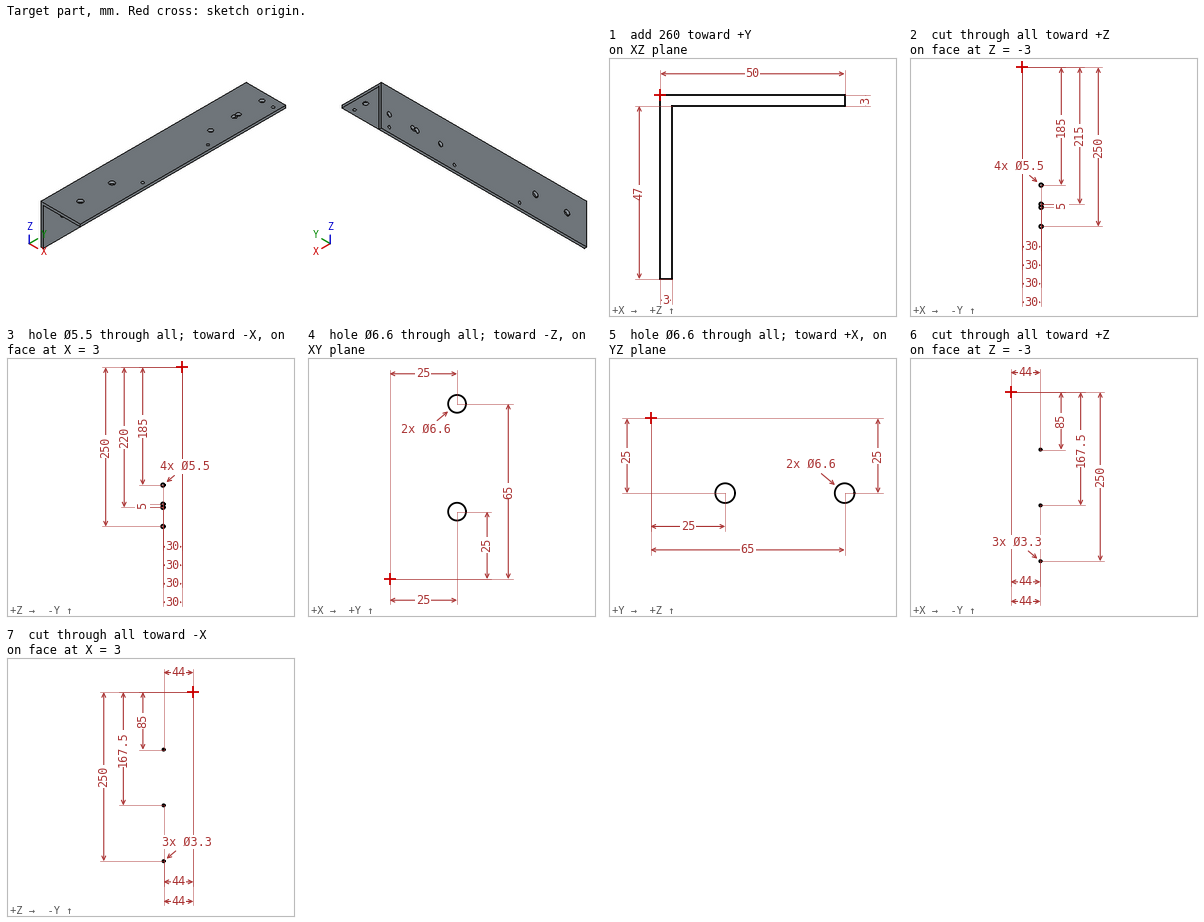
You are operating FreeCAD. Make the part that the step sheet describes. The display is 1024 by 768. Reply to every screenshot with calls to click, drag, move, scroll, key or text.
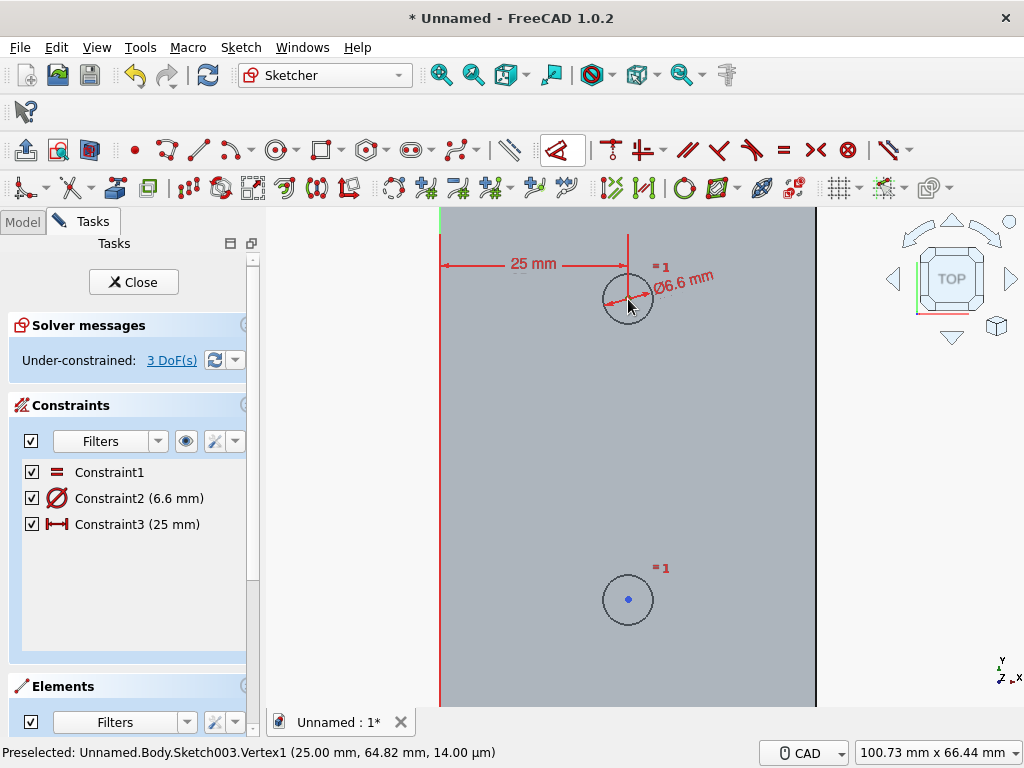
key(i)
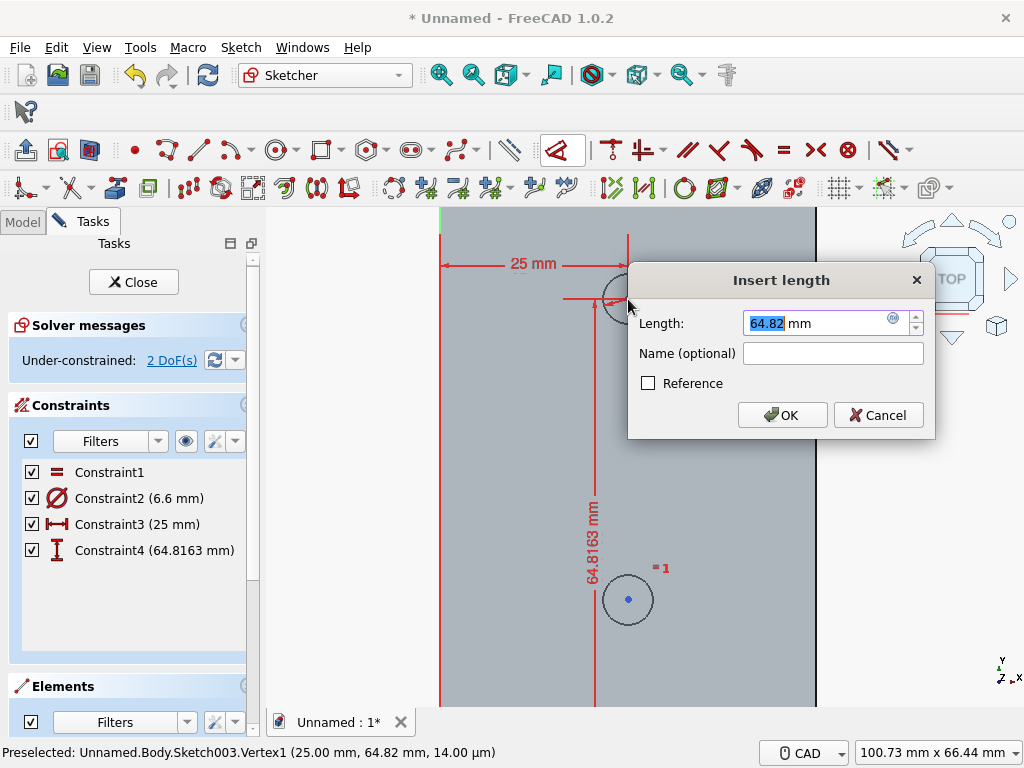
text(65)
key(Return)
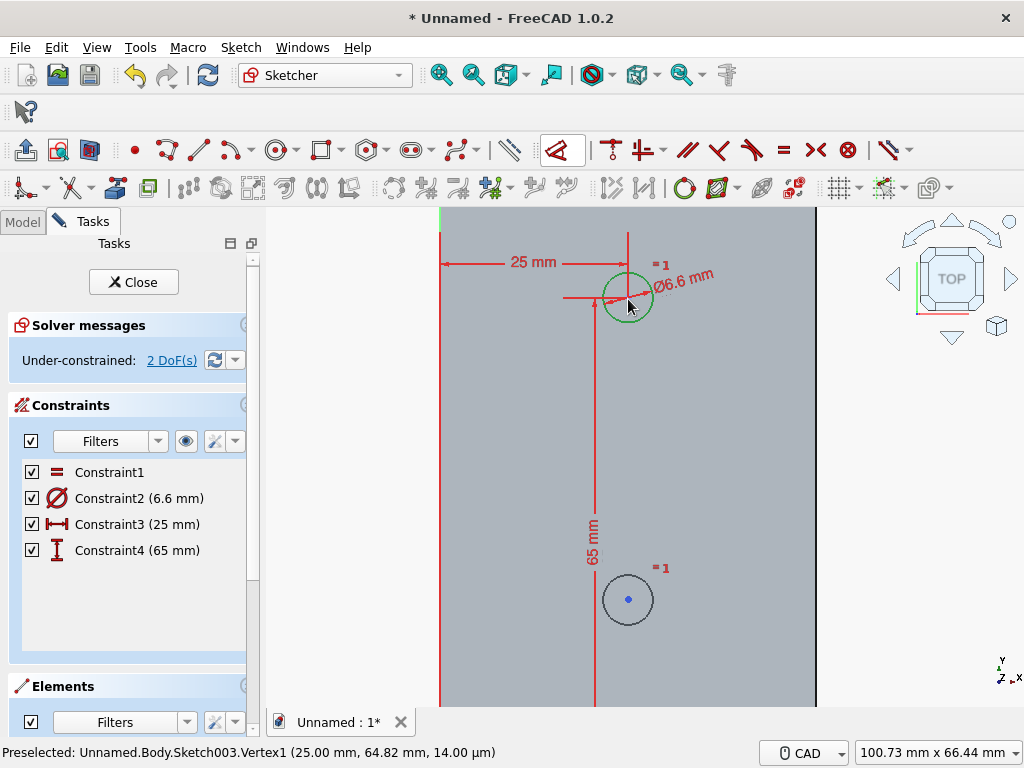
click(628, 600)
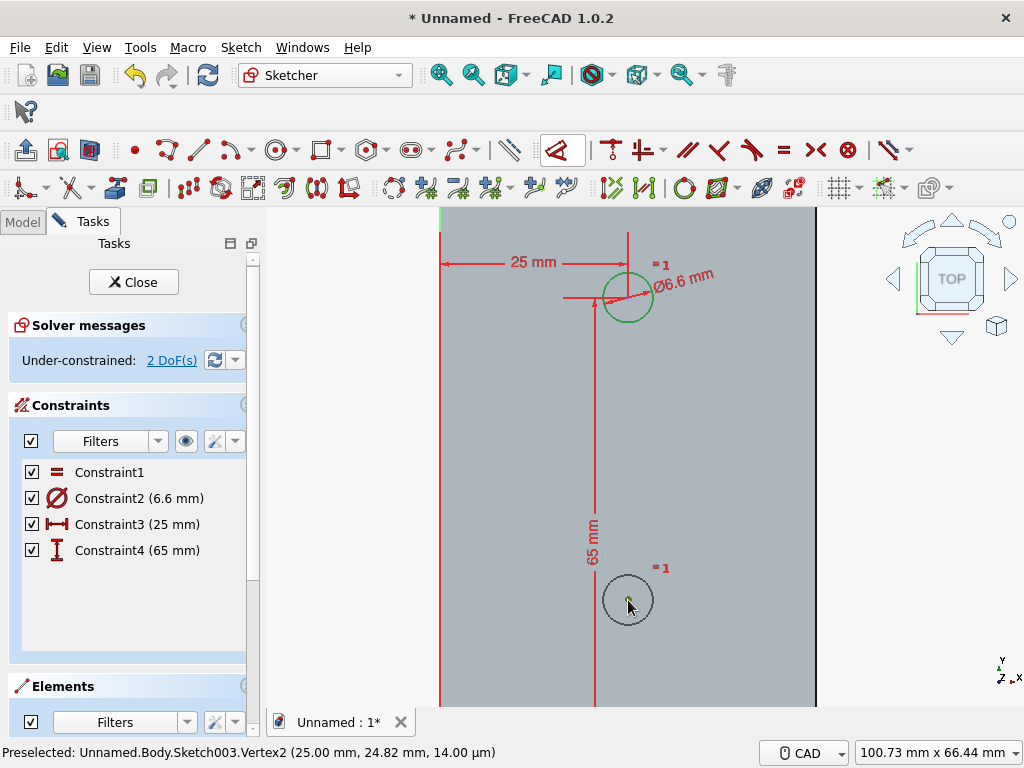
key(l)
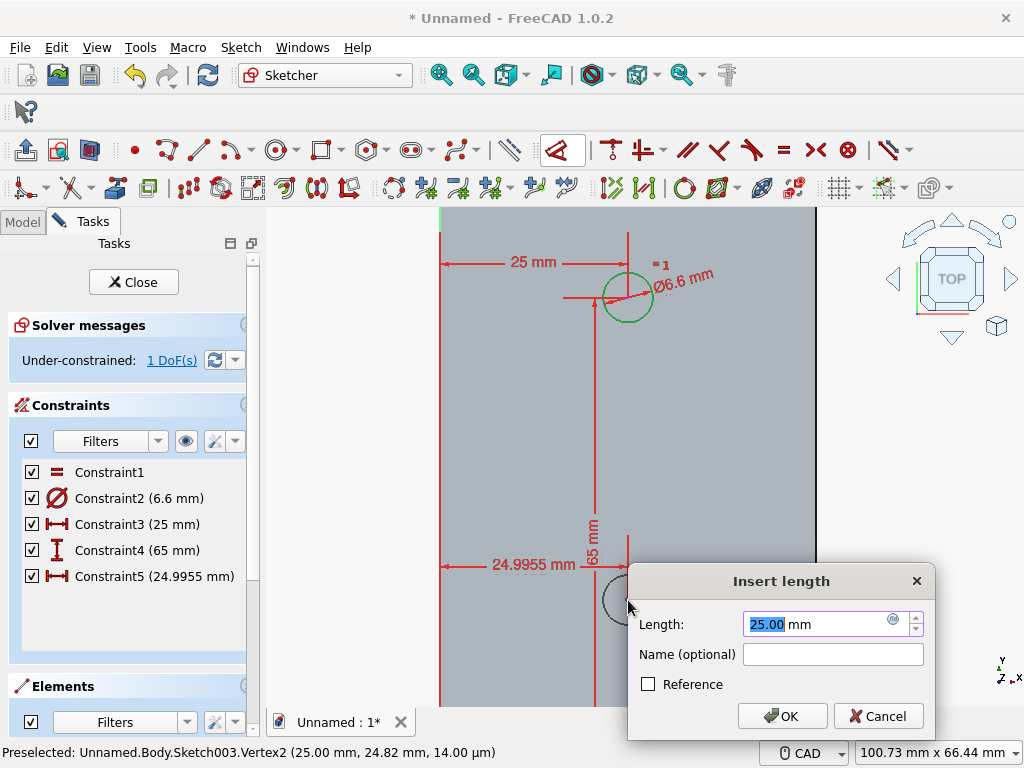
text(25)
key(Return)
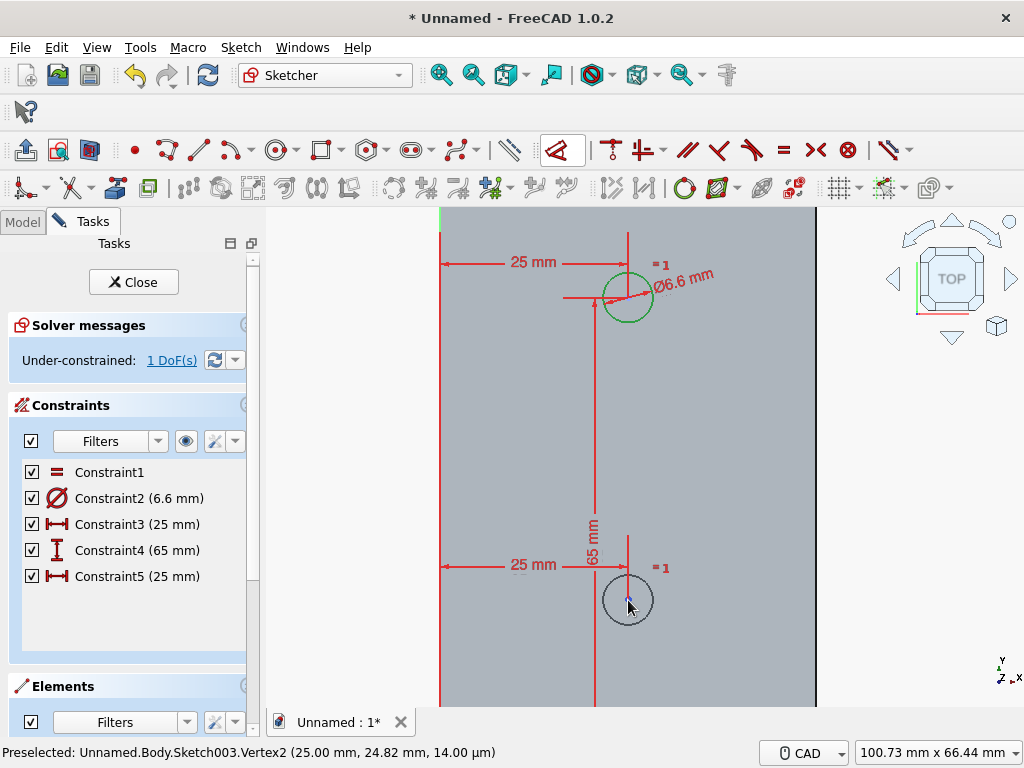
click(628, 600)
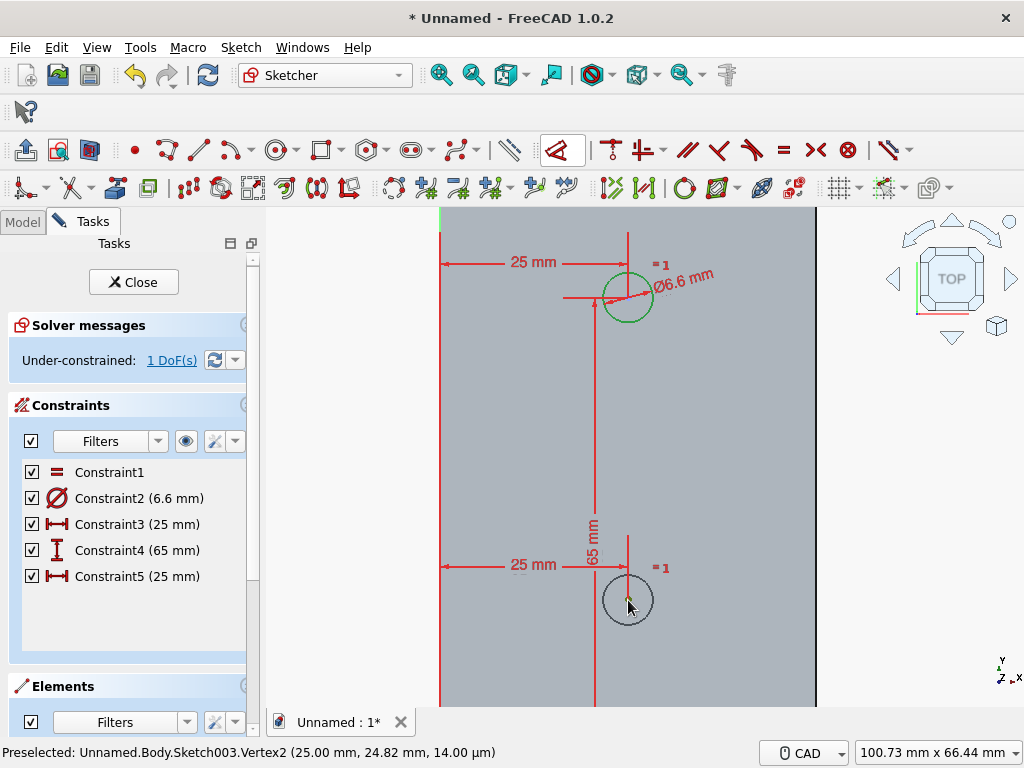
key(i)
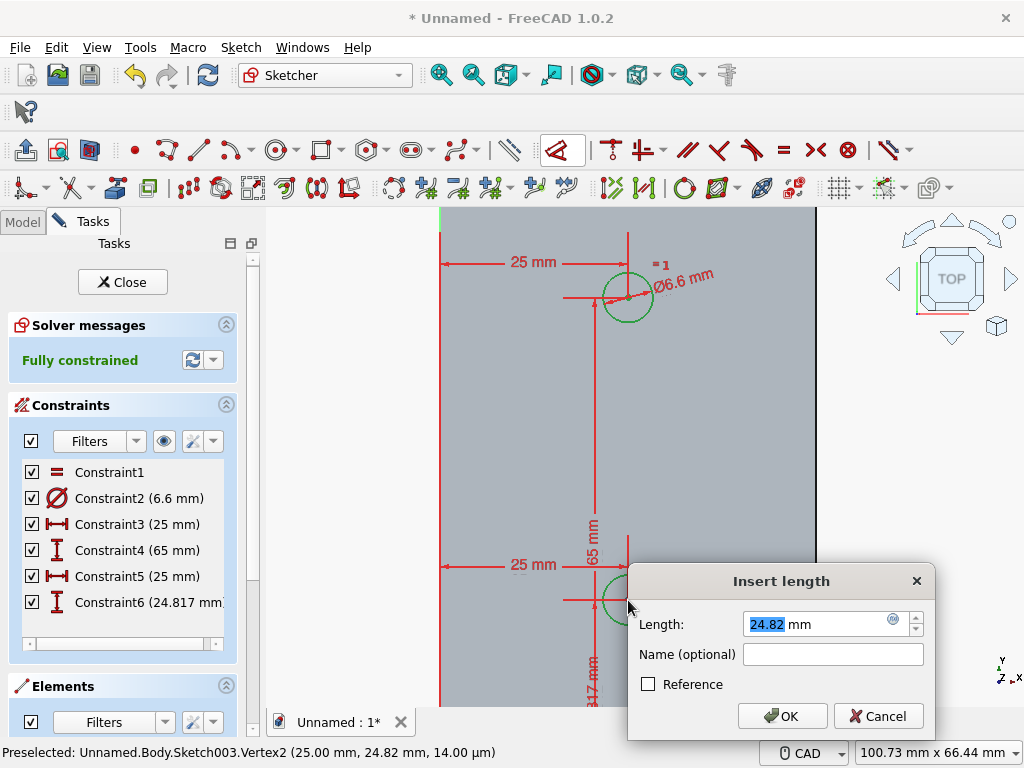
text(25)
key(Return)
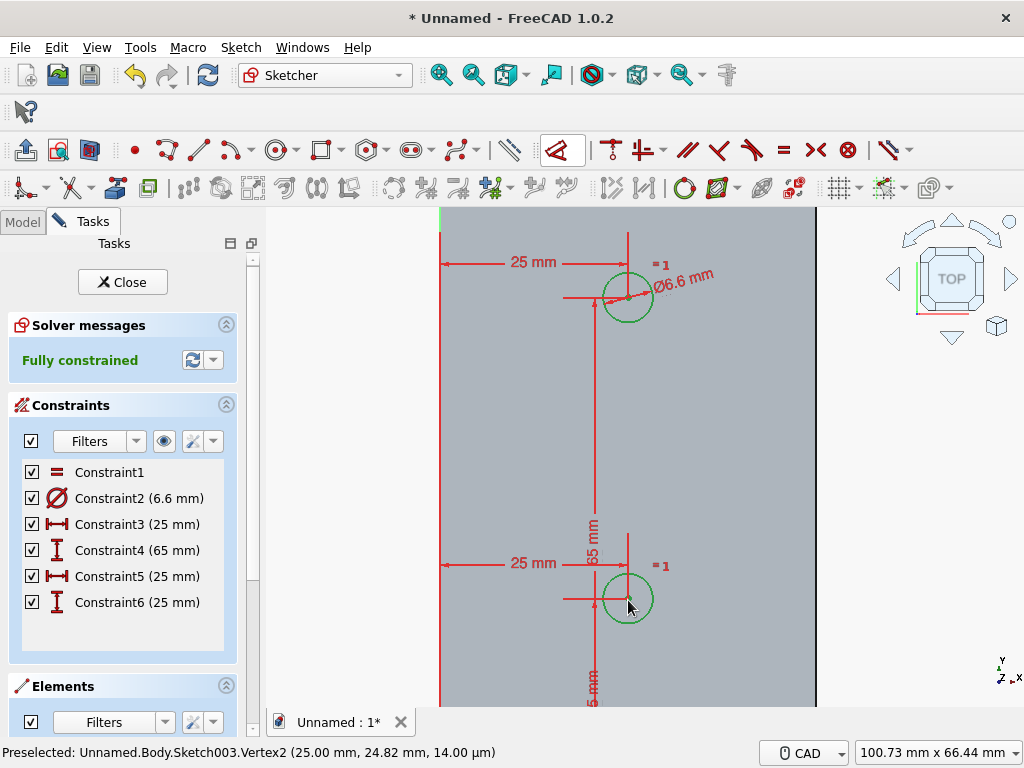
click(123, 282)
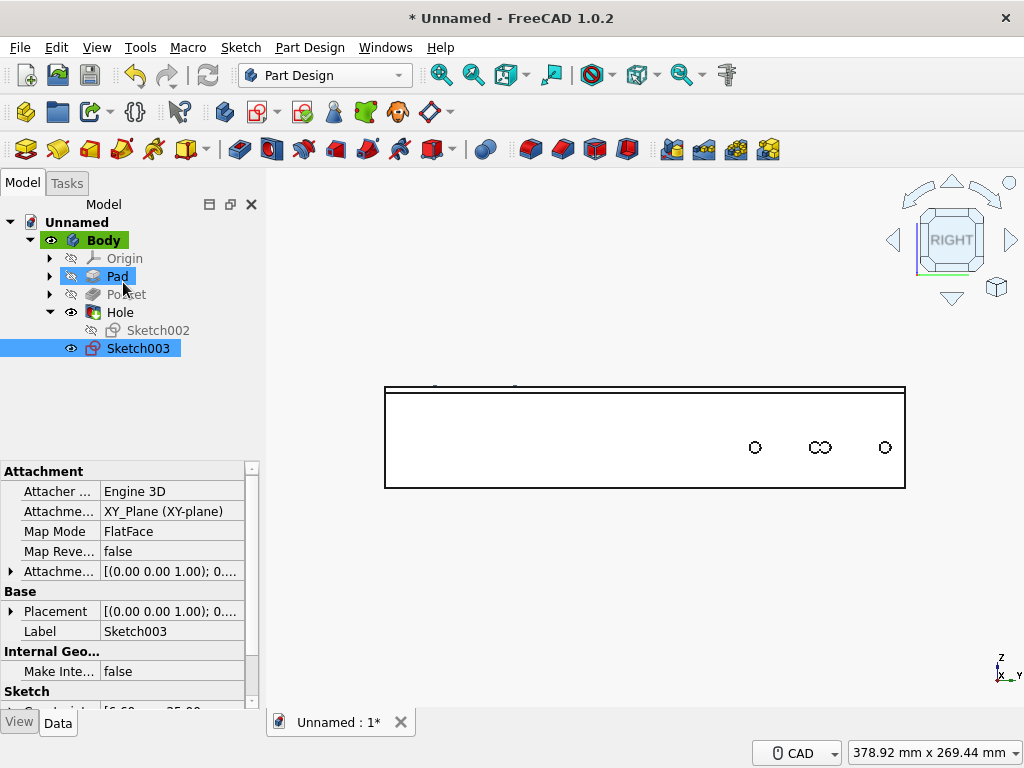
click(272, 150)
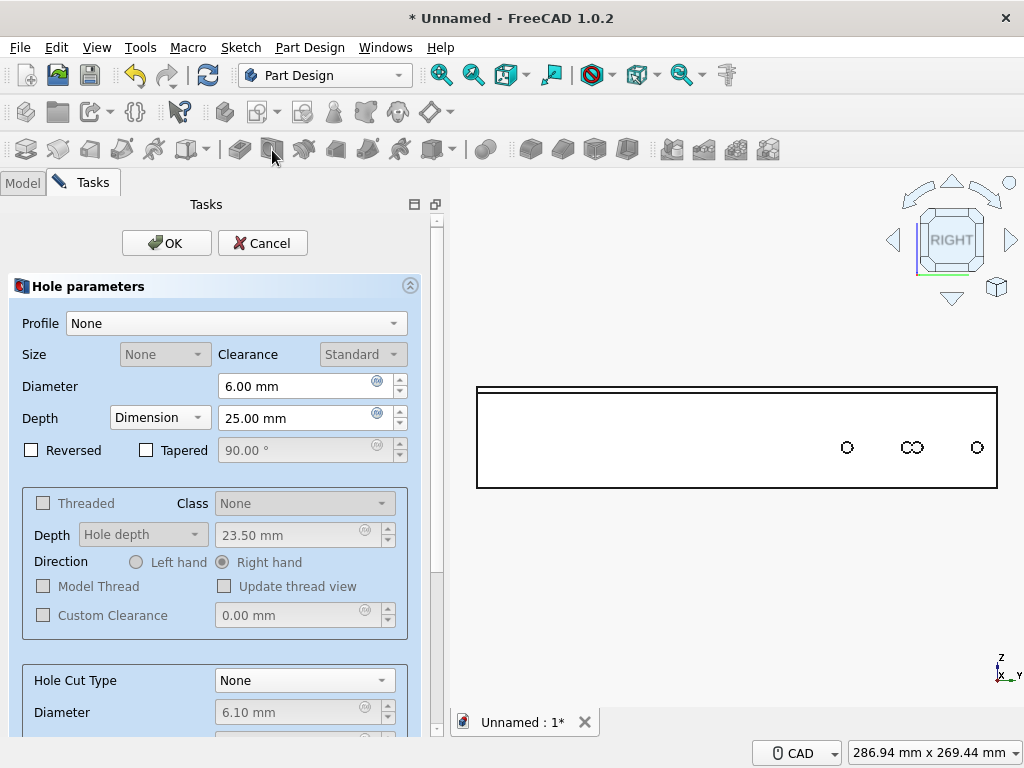
triple_click(305, 386)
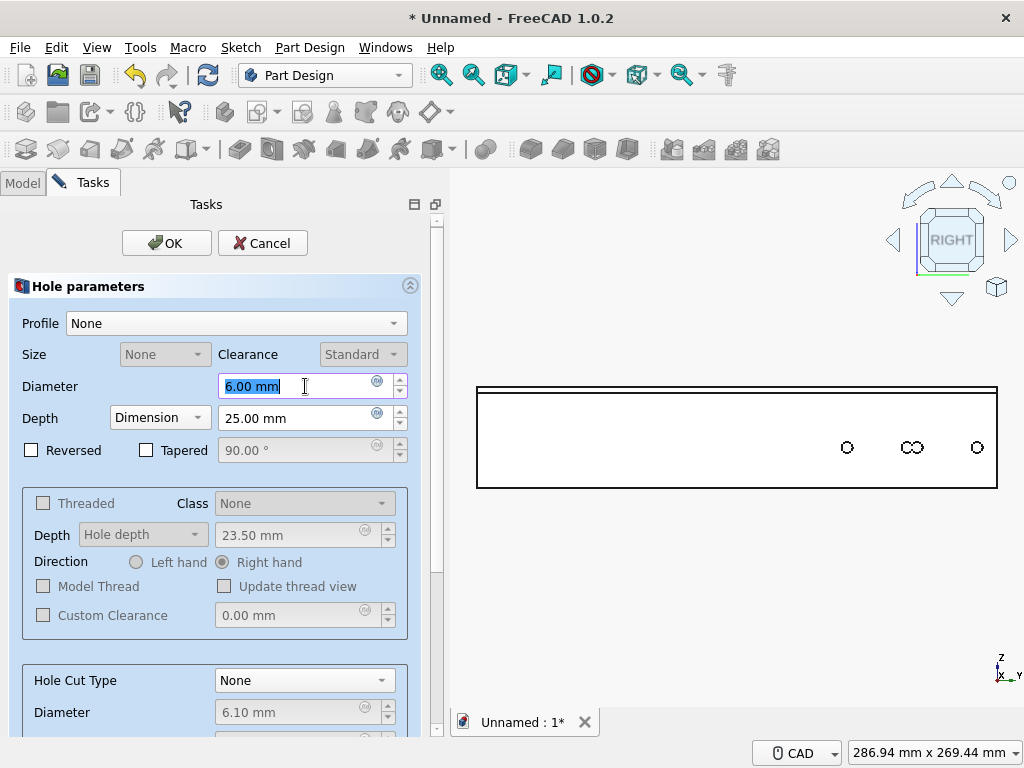
text(6.6)
key(Tab)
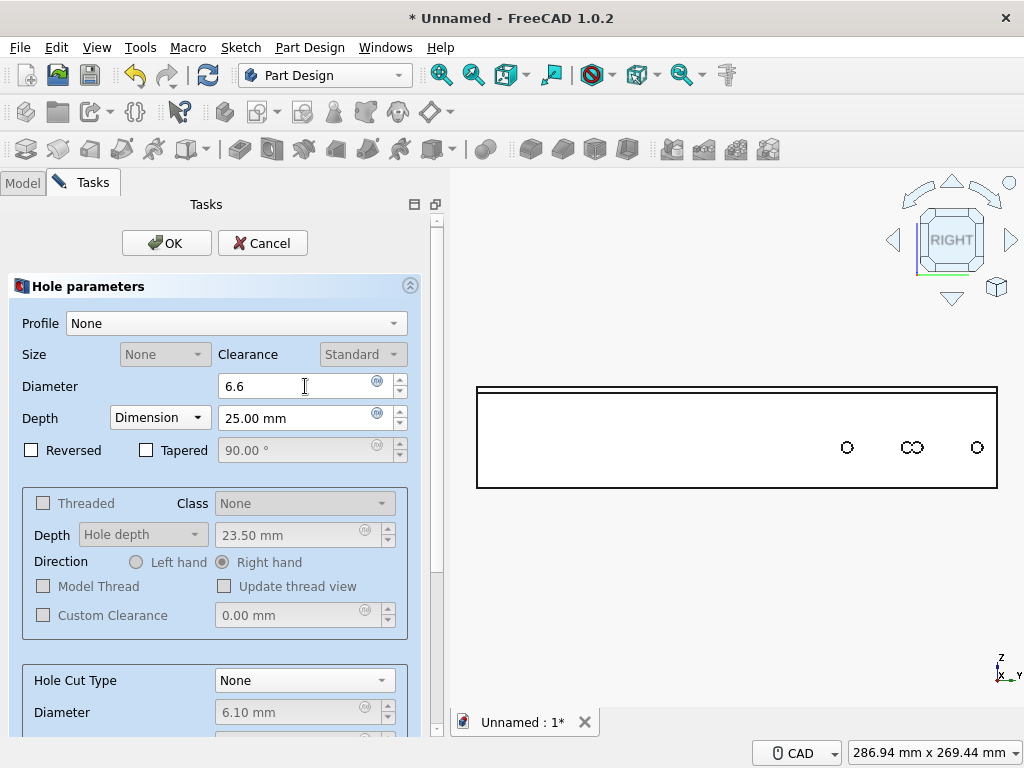
click(161, 418)